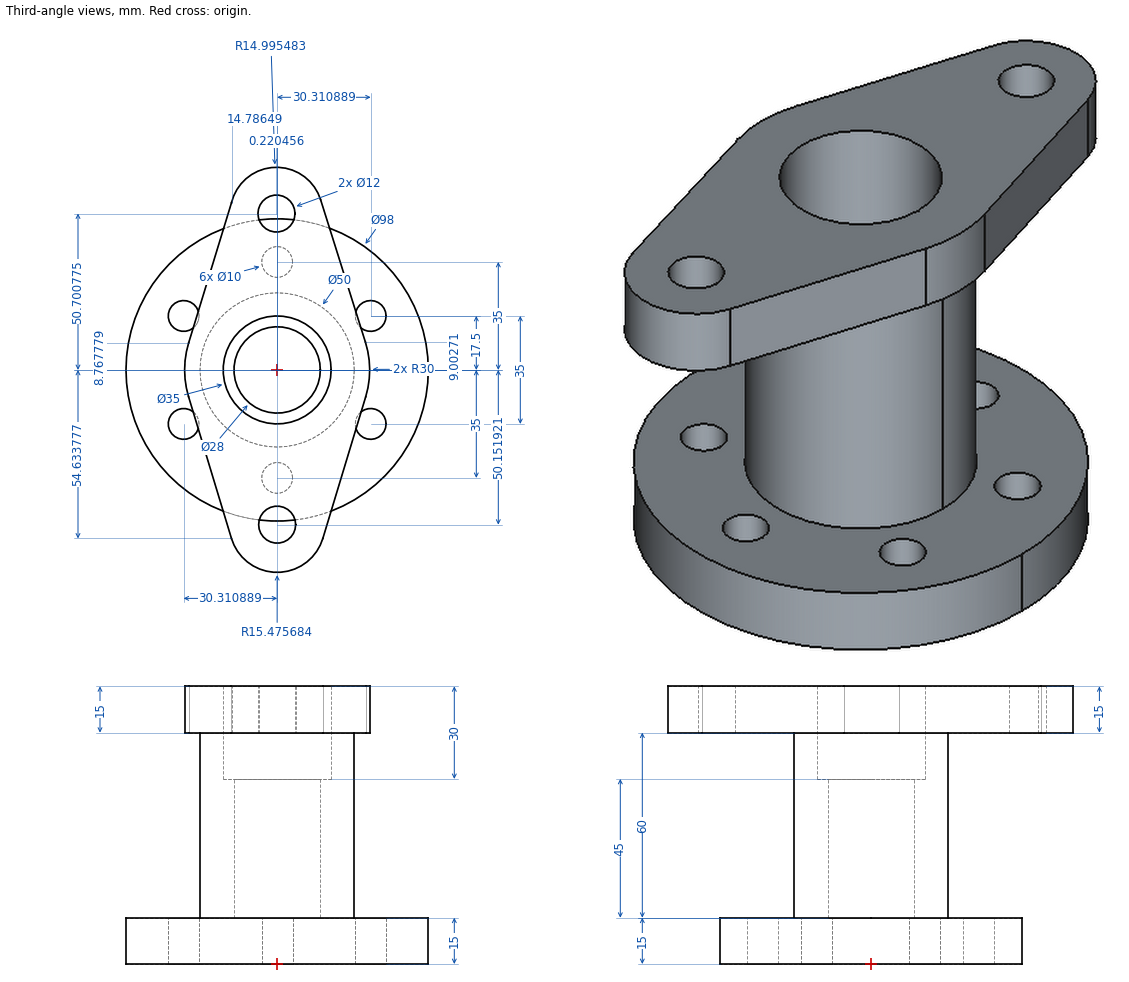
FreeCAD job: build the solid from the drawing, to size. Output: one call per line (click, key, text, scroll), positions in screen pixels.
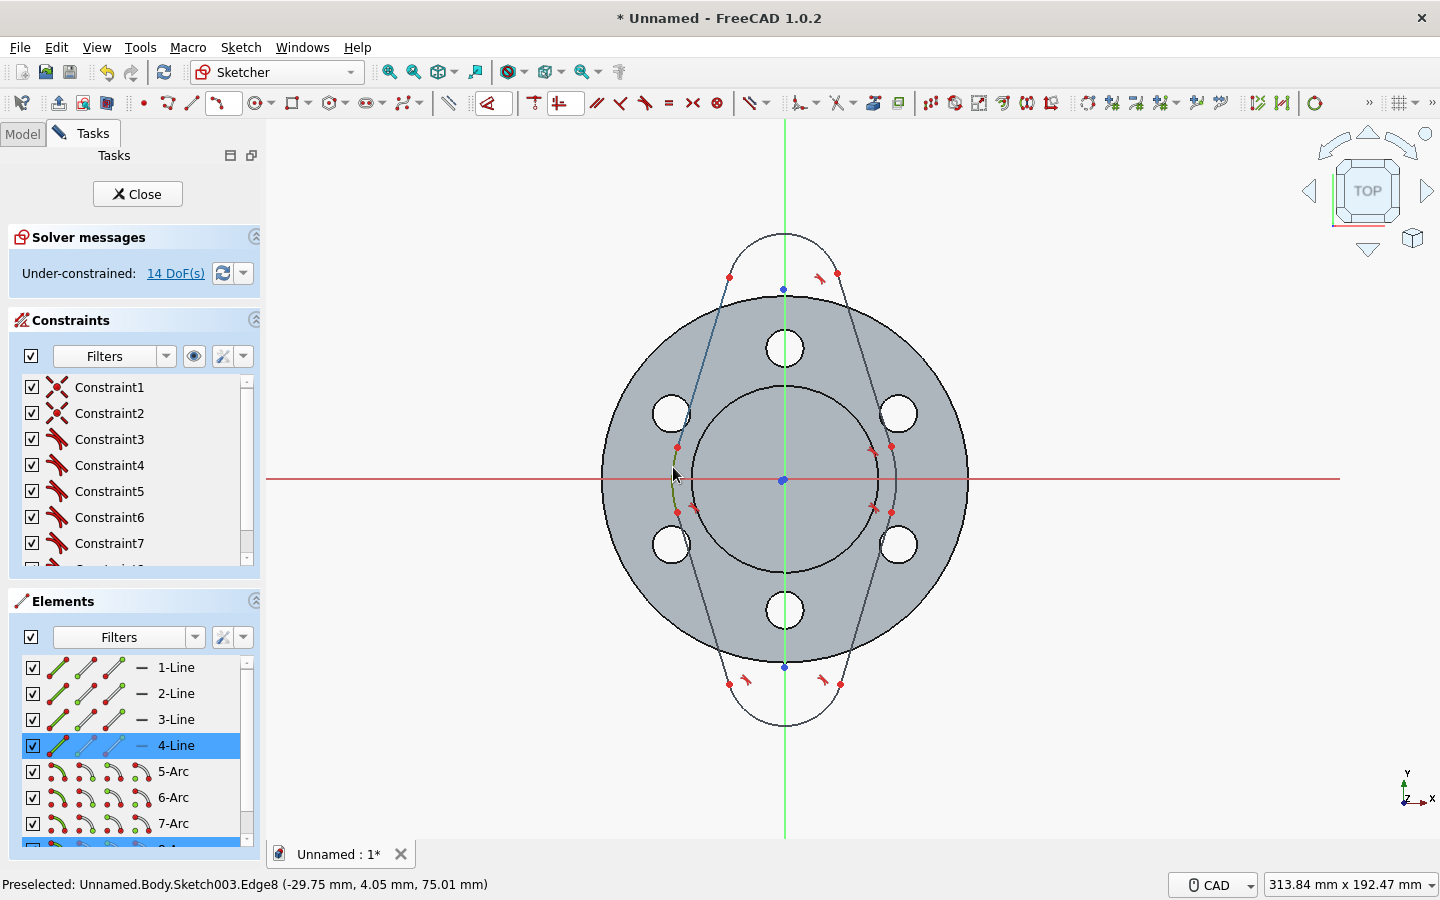
click(646, 104)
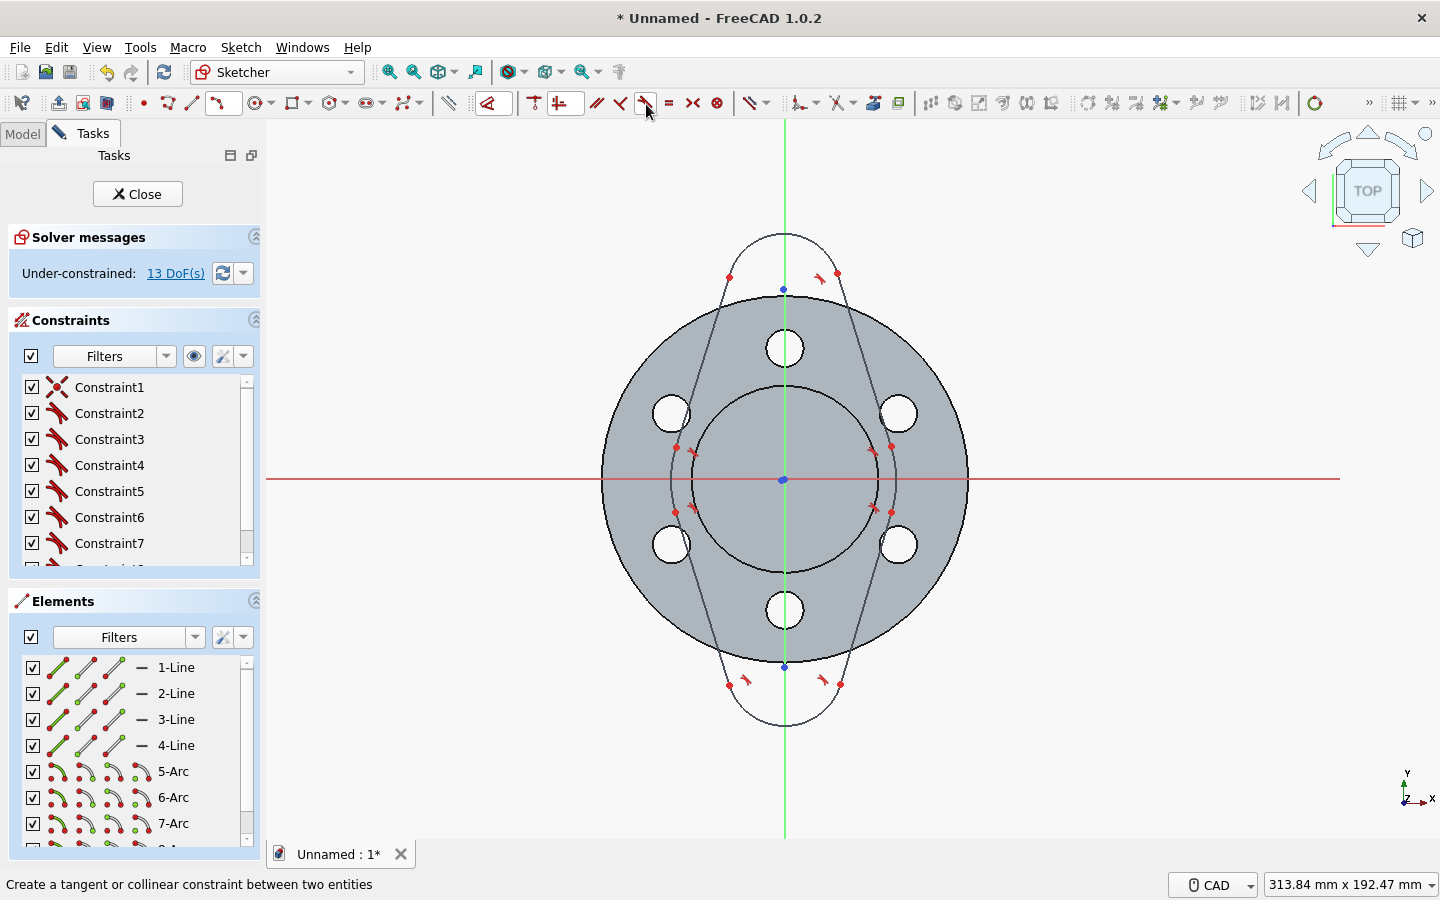
click(895, 493)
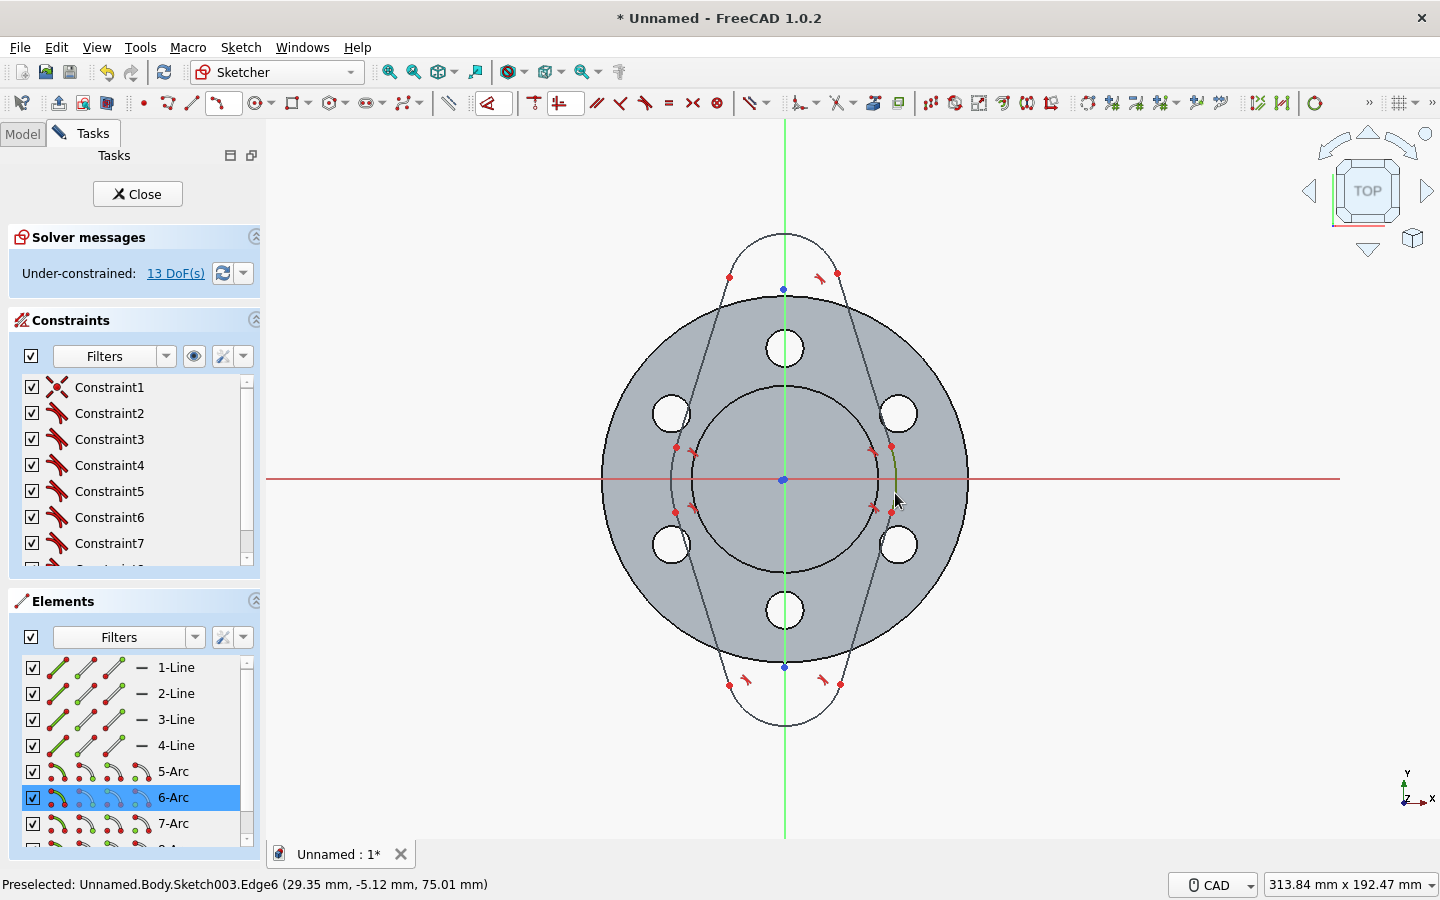
click(672, 467)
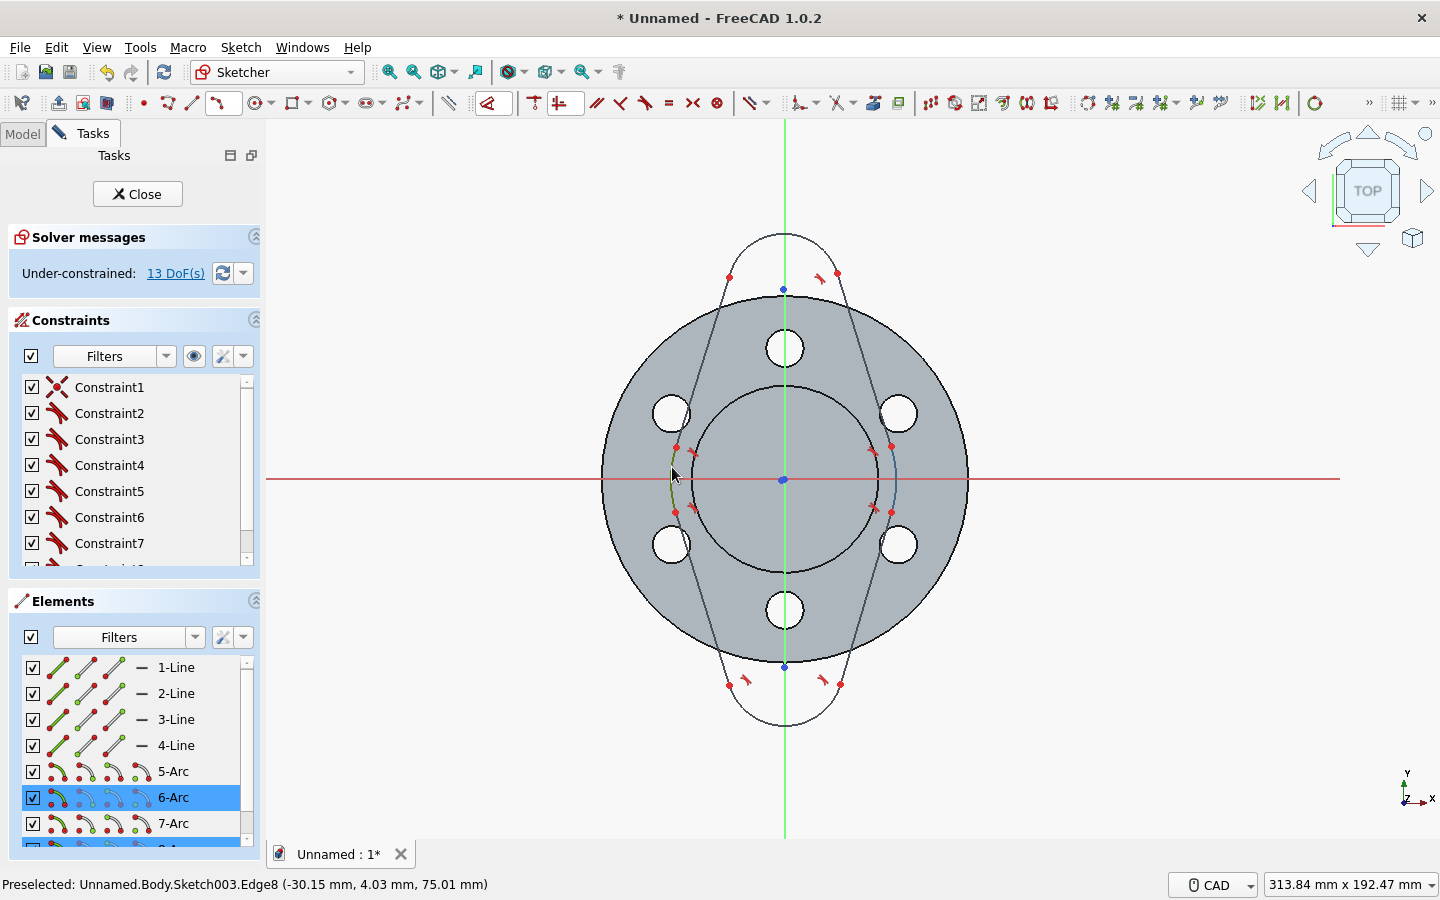
key(c)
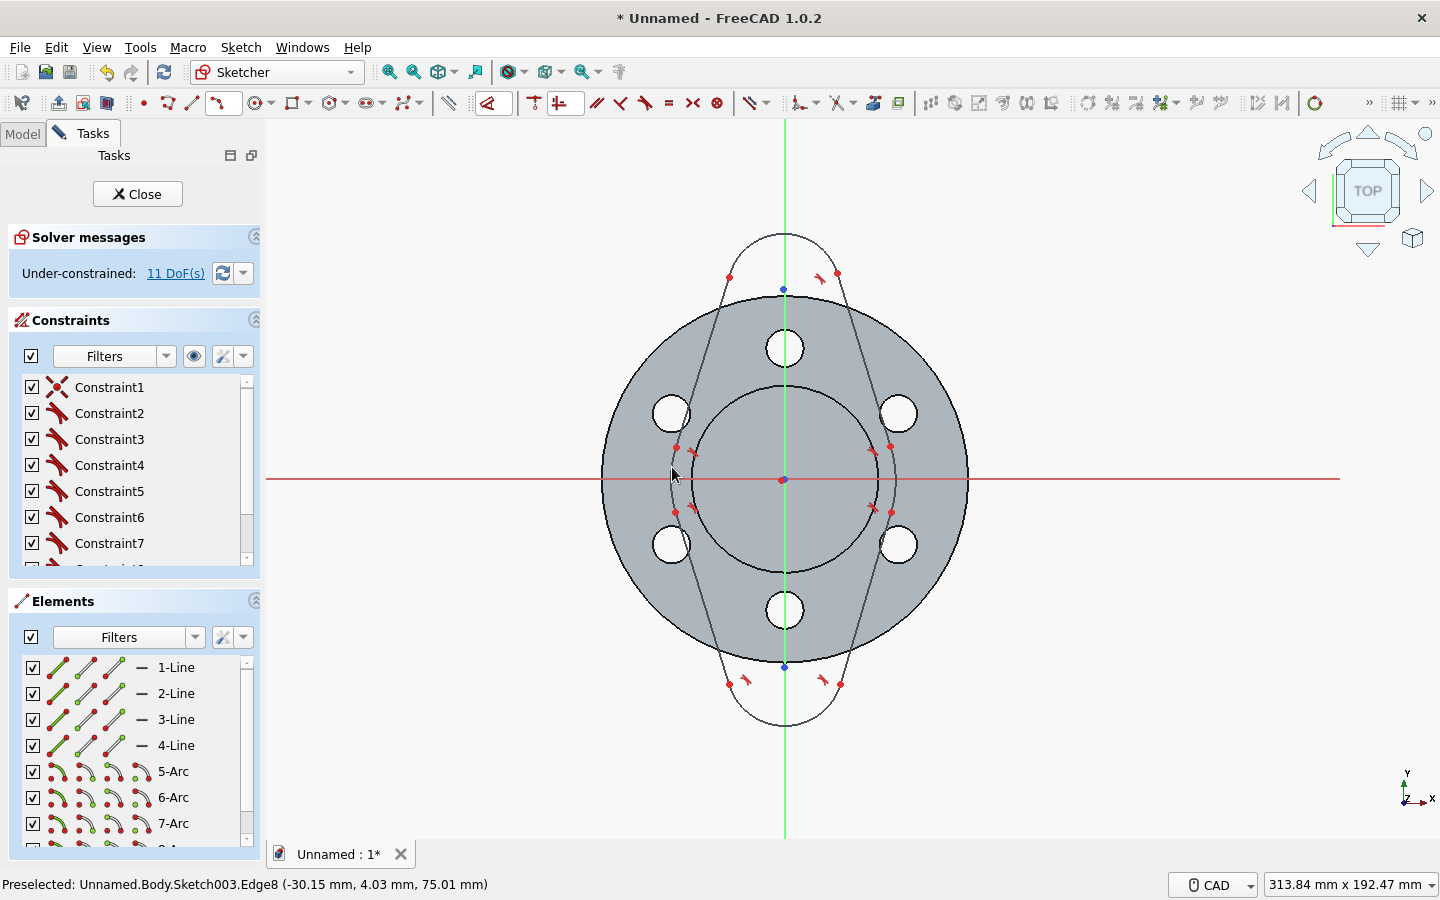
drag(771, 469, 795, 490)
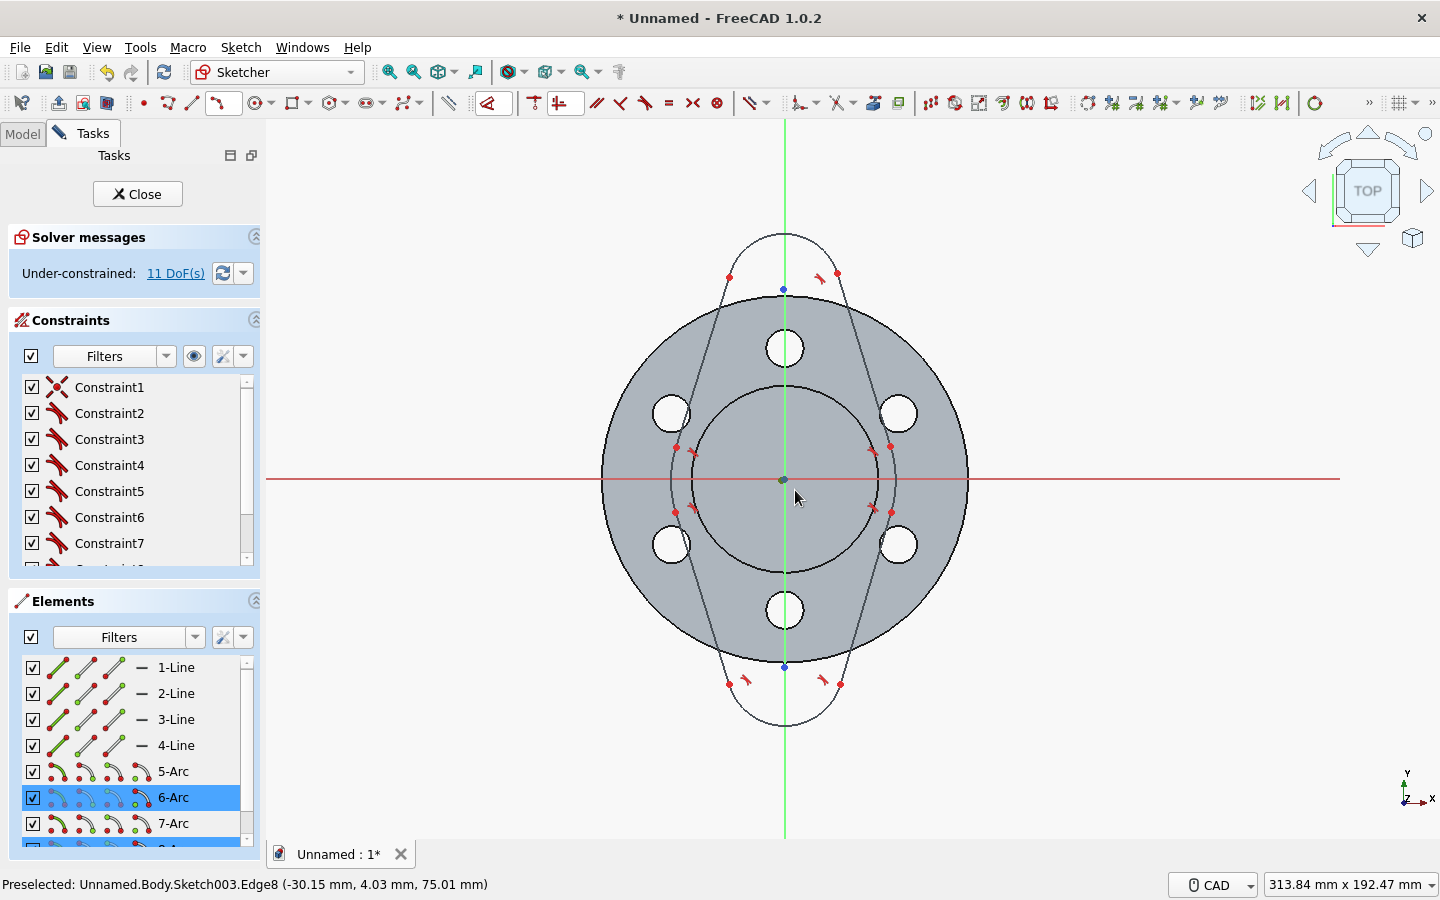
key(c)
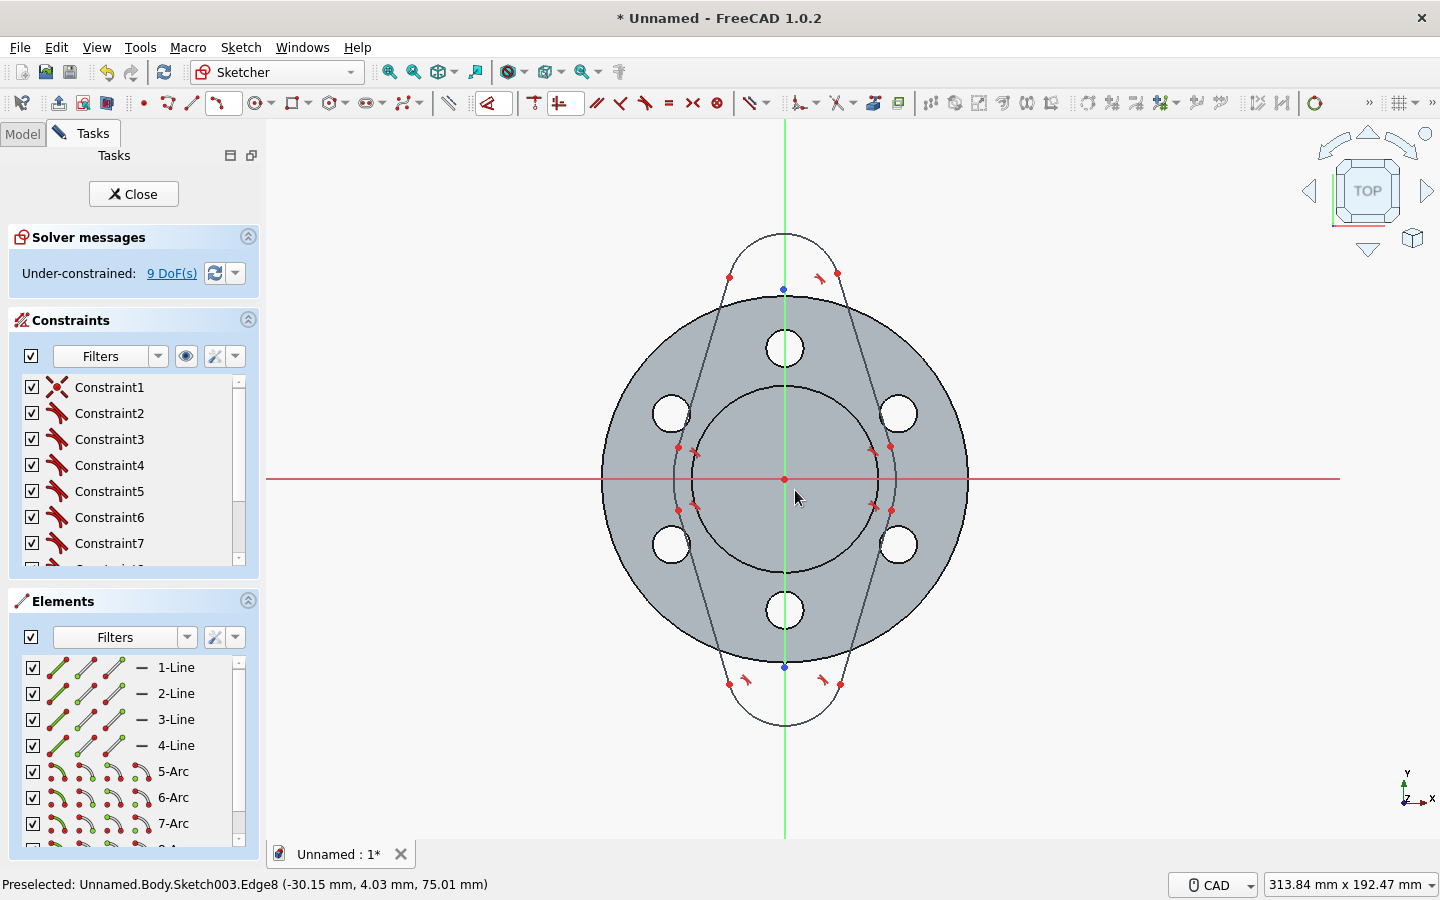
click(895, 491)